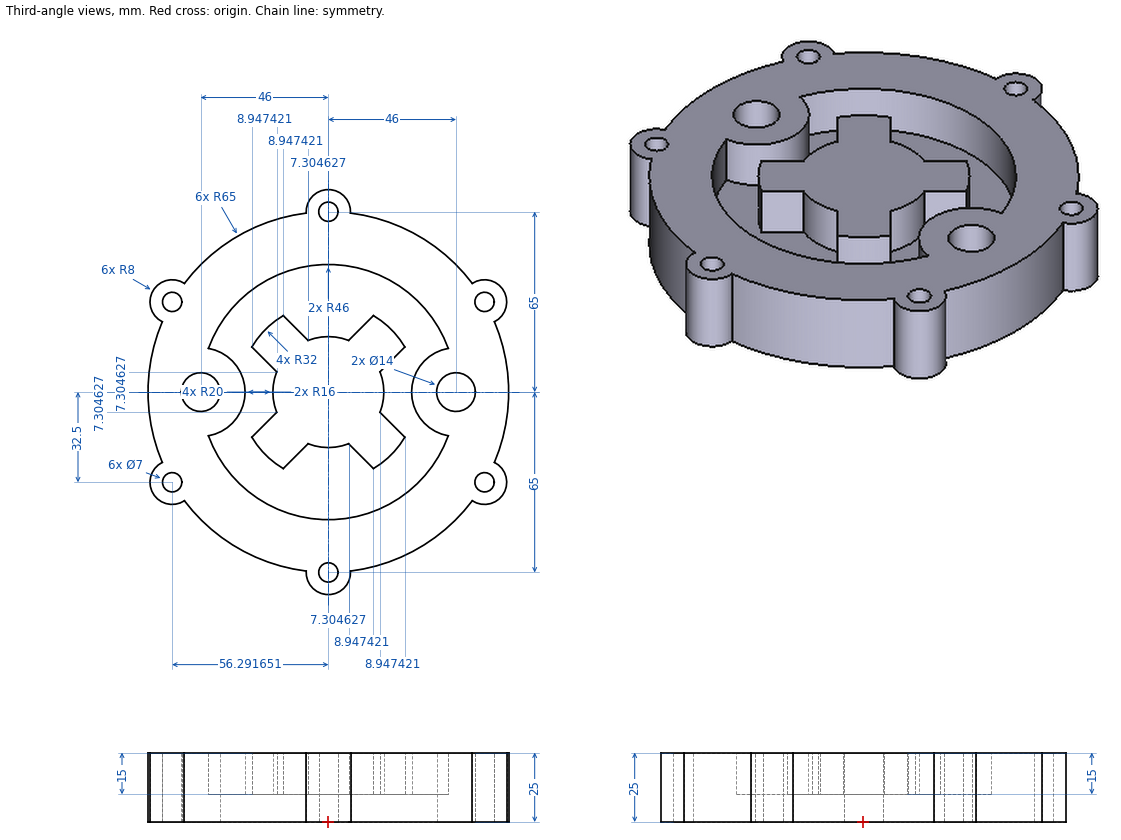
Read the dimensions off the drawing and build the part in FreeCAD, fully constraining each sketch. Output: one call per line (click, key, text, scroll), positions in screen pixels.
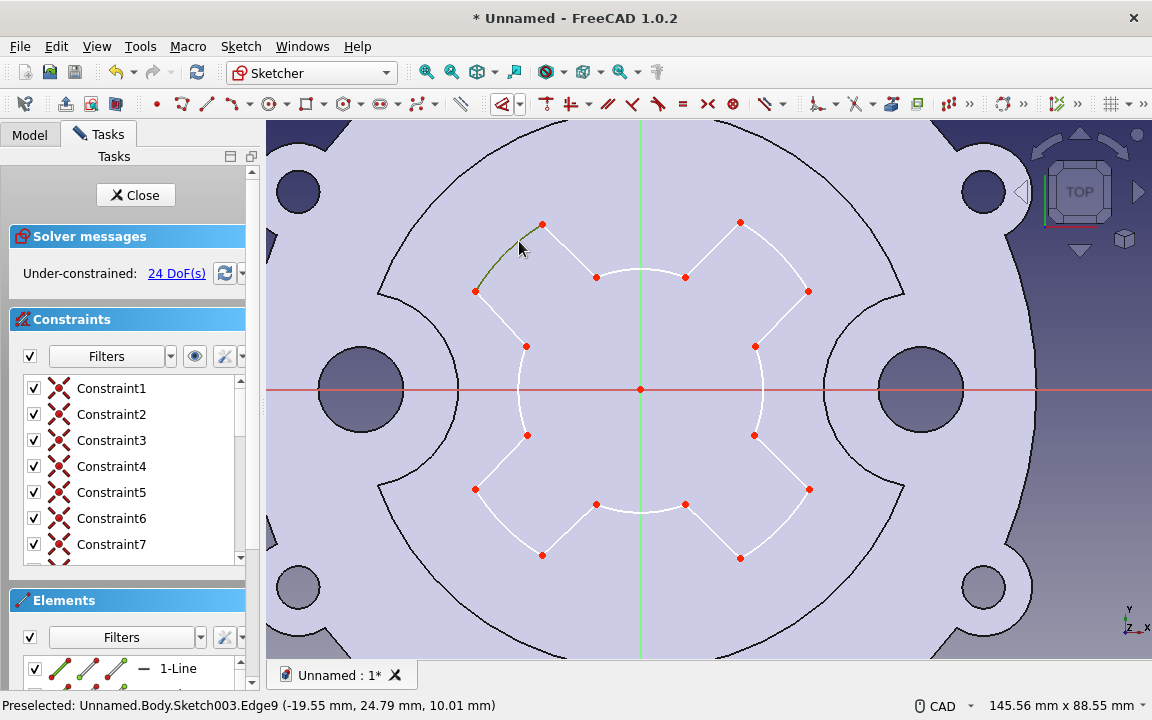
click(492, 513)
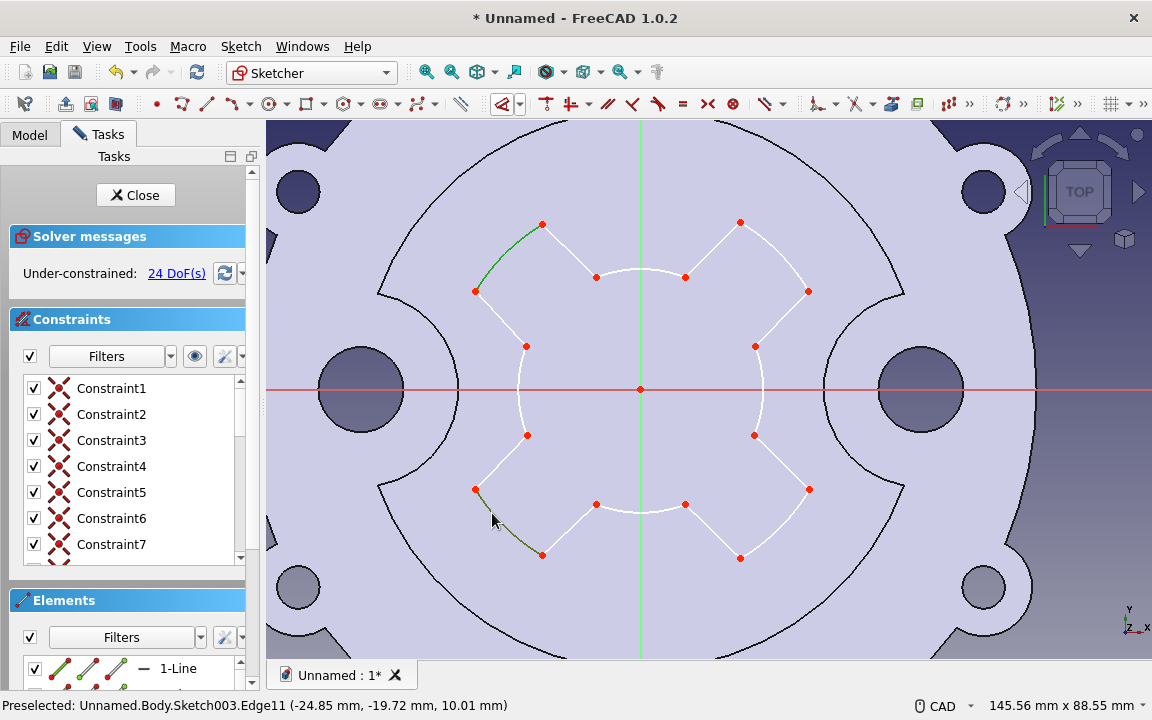
click(765, 542)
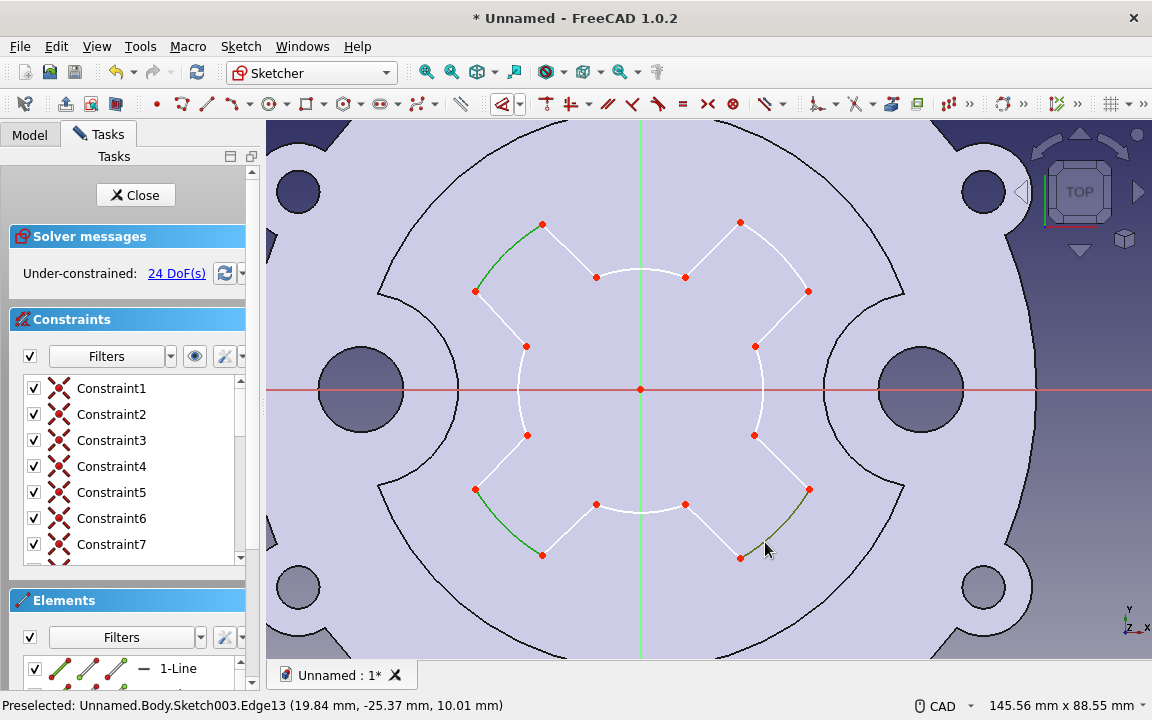
click(792, 267)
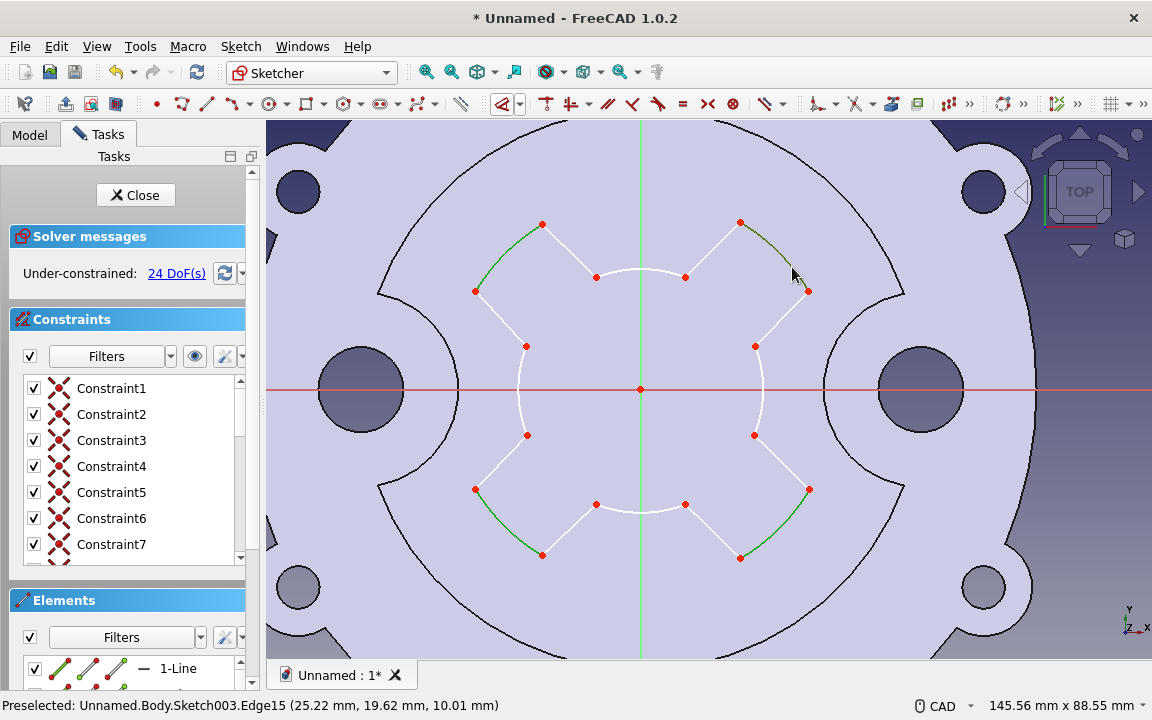
click(683, 104)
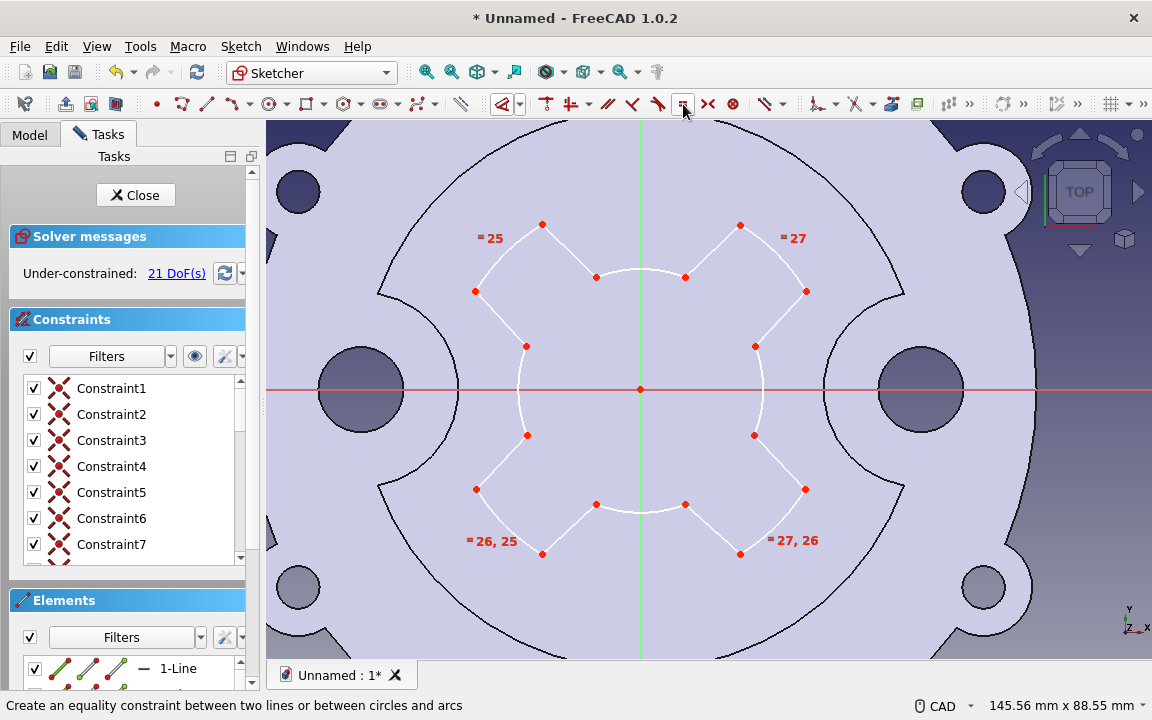
click(520, 373)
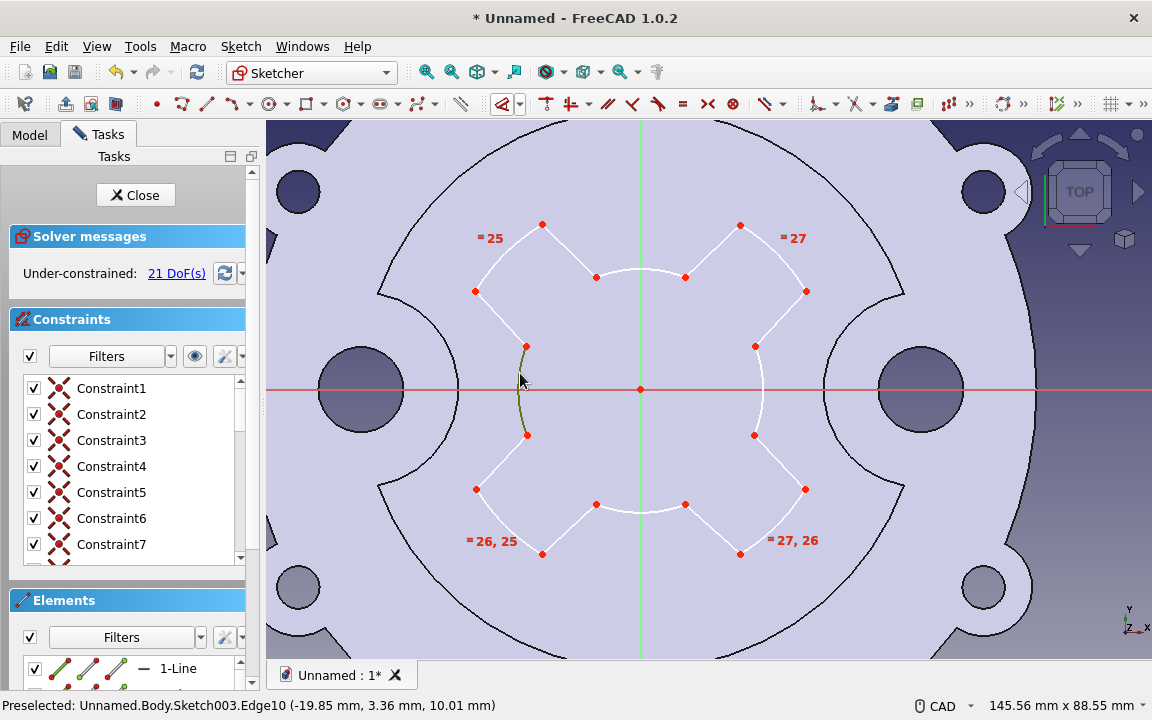
click(623, 511)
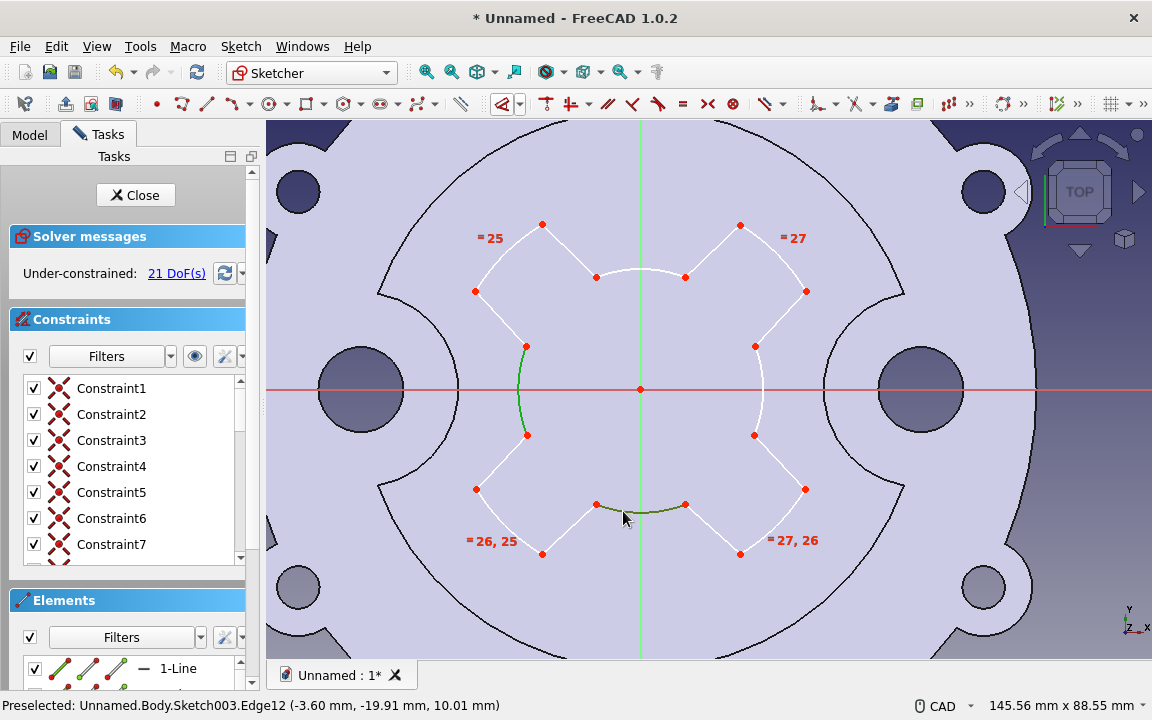
click(762, 409)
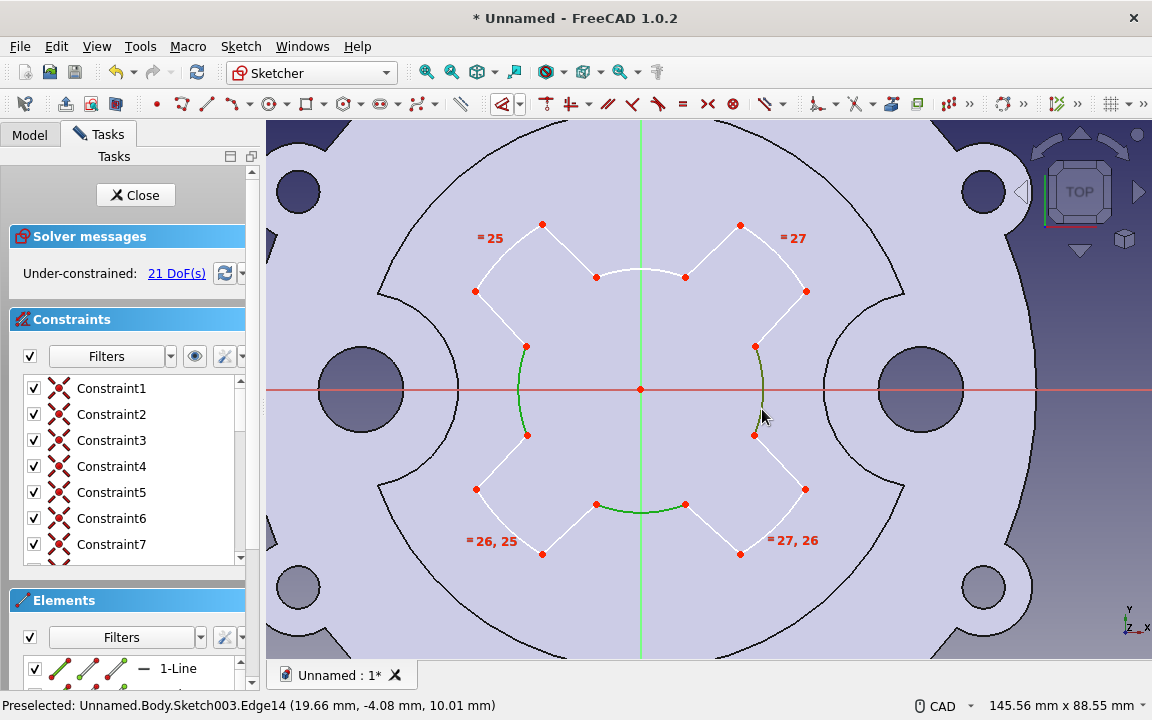
click(659, 270)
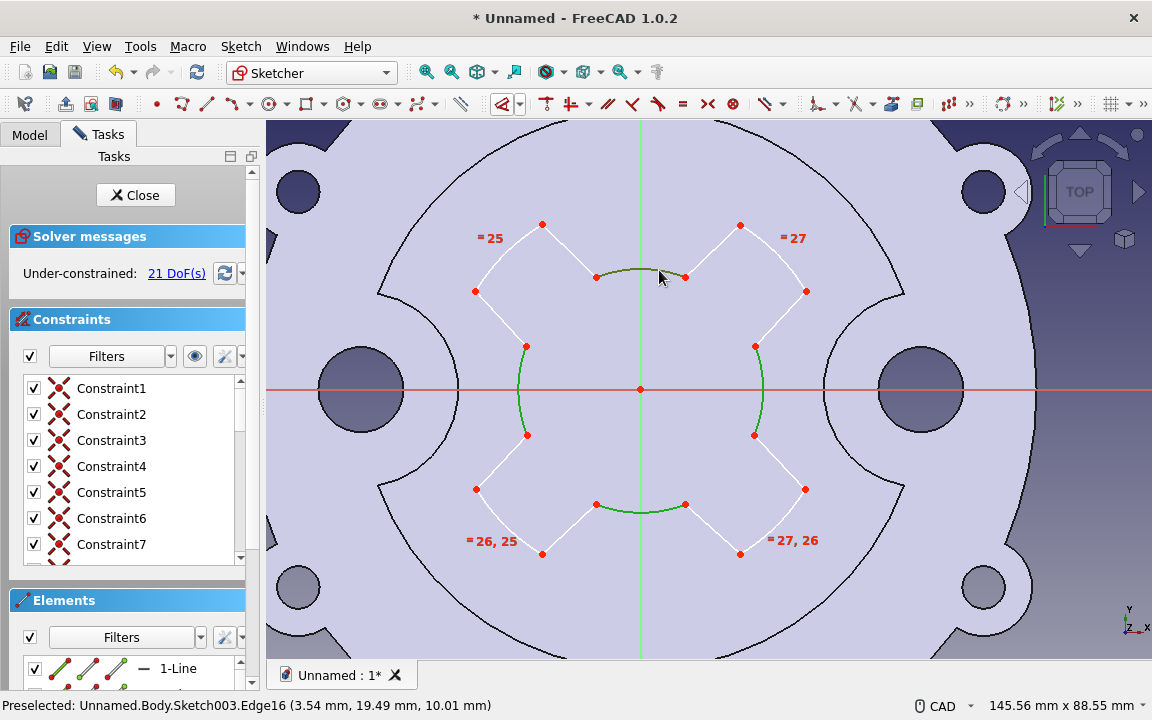
click(683, 104)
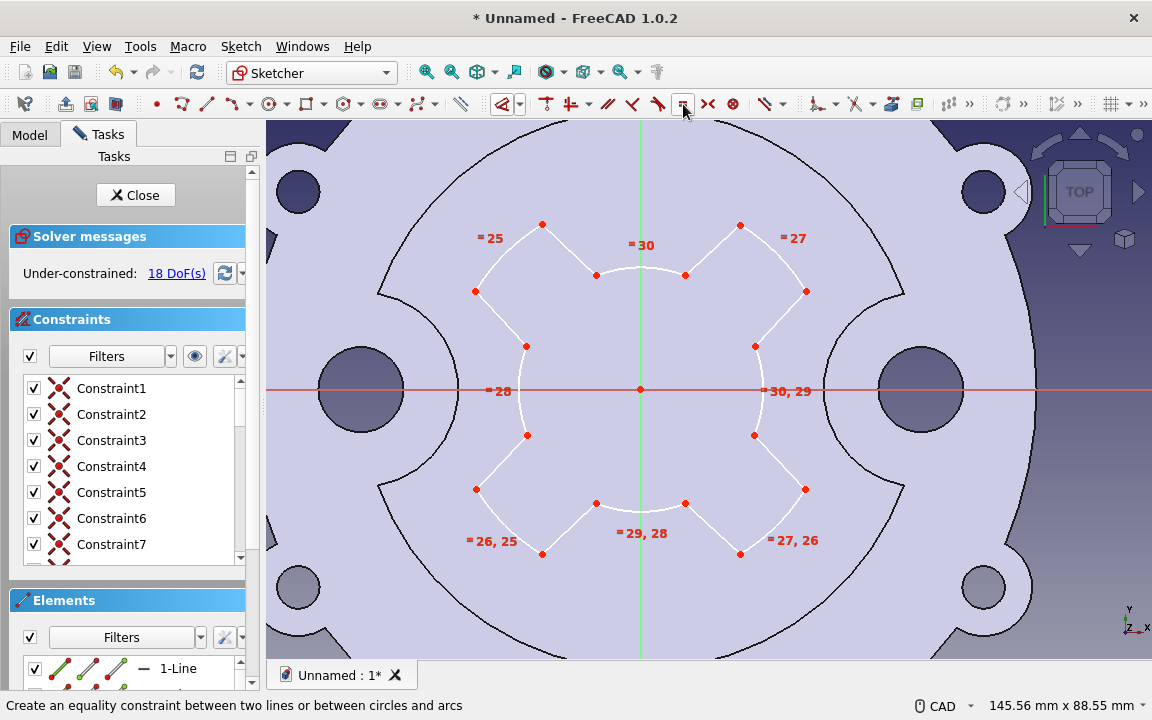
click(519, 241)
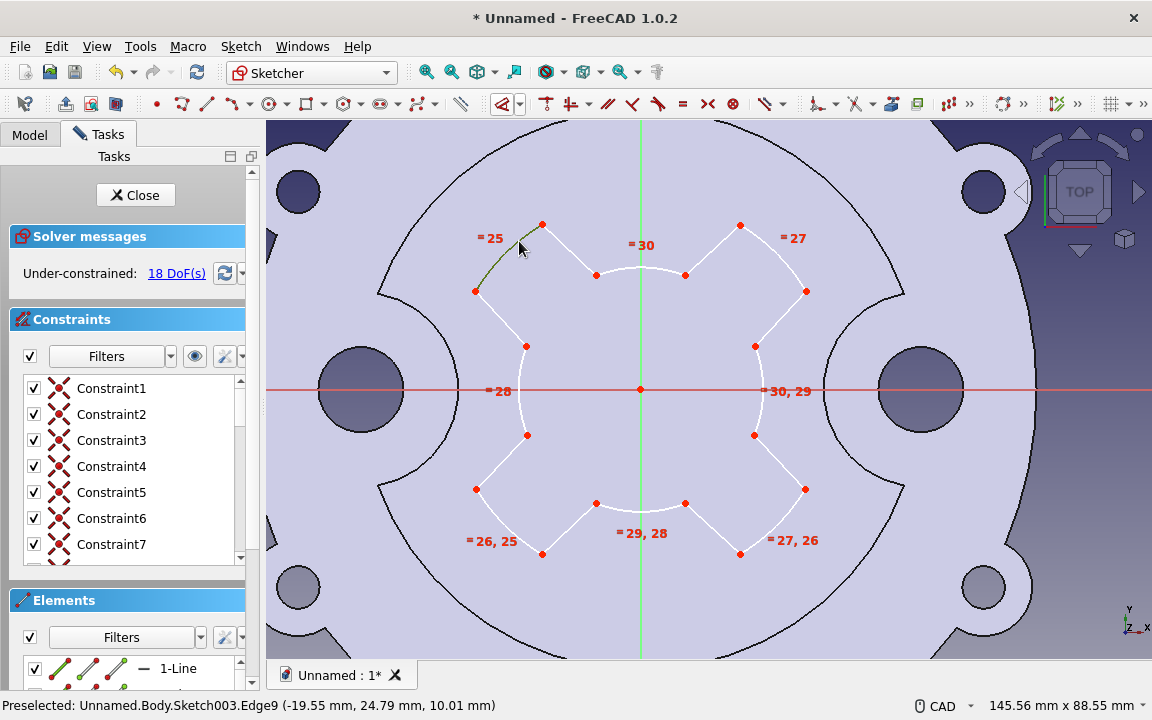
key(k)
key(r)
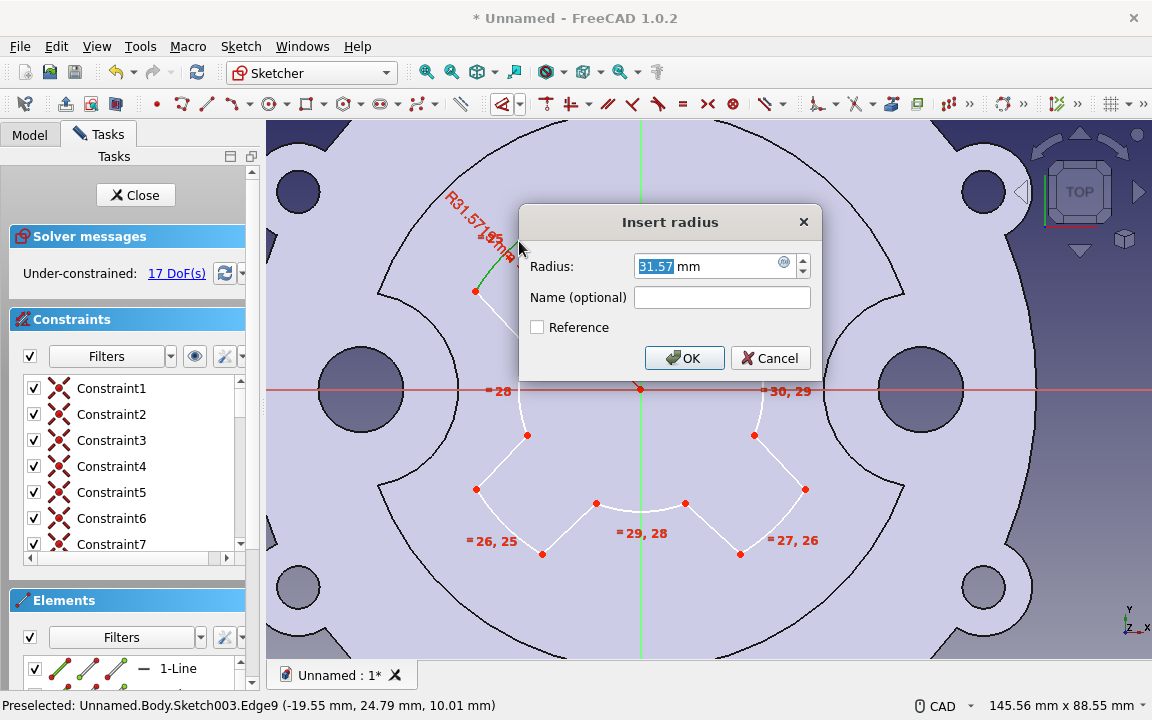
text(32)
key(Return)